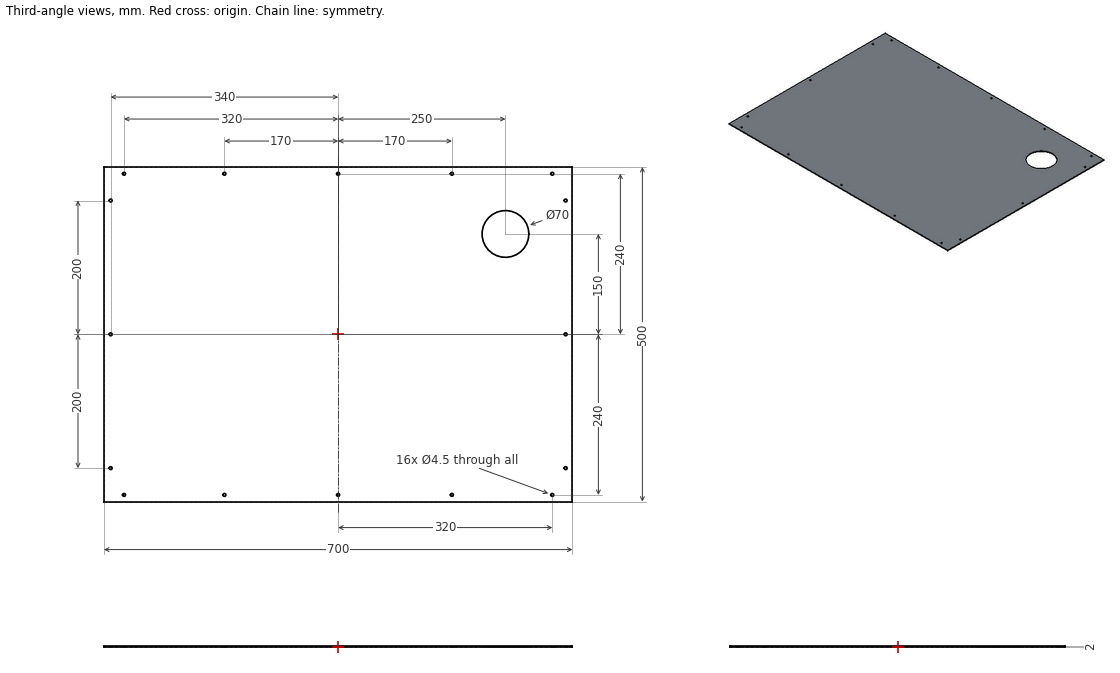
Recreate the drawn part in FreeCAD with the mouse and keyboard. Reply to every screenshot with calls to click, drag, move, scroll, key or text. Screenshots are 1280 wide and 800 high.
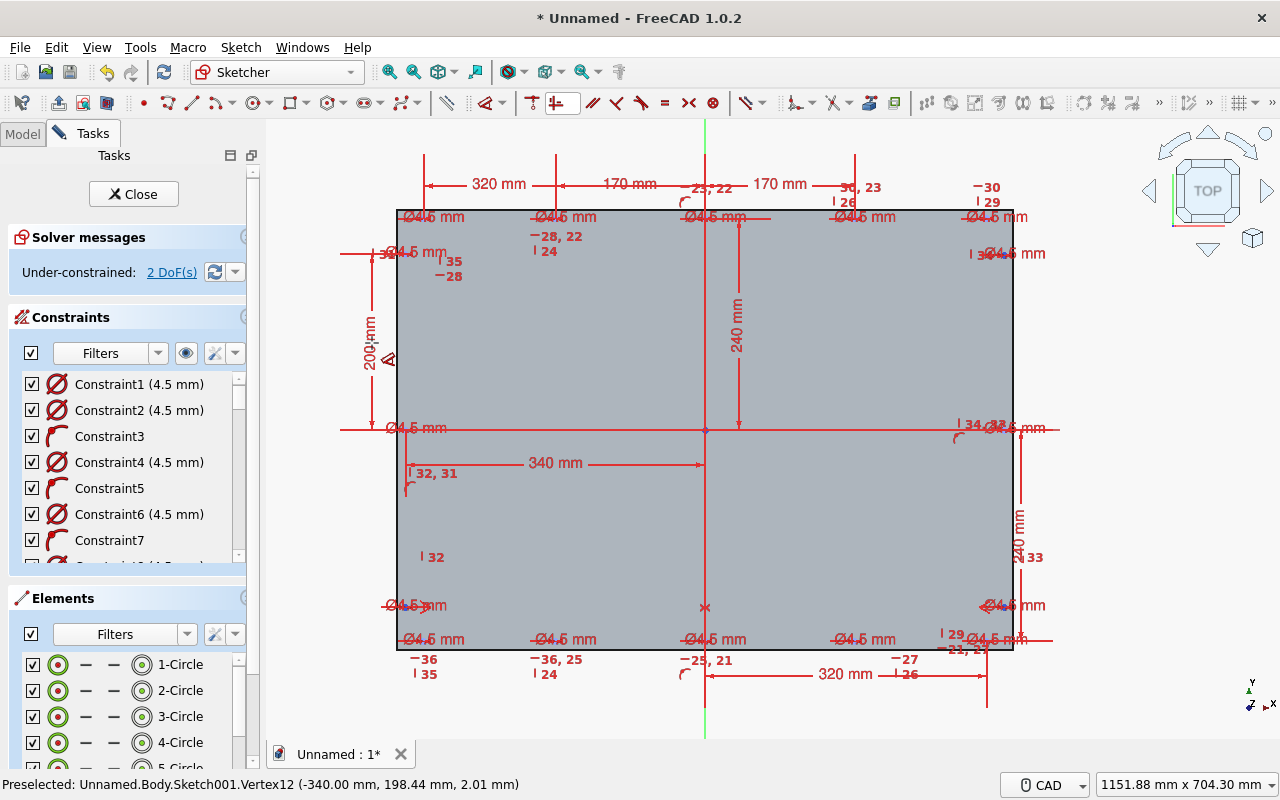
click(406, 607)
click(372, 519)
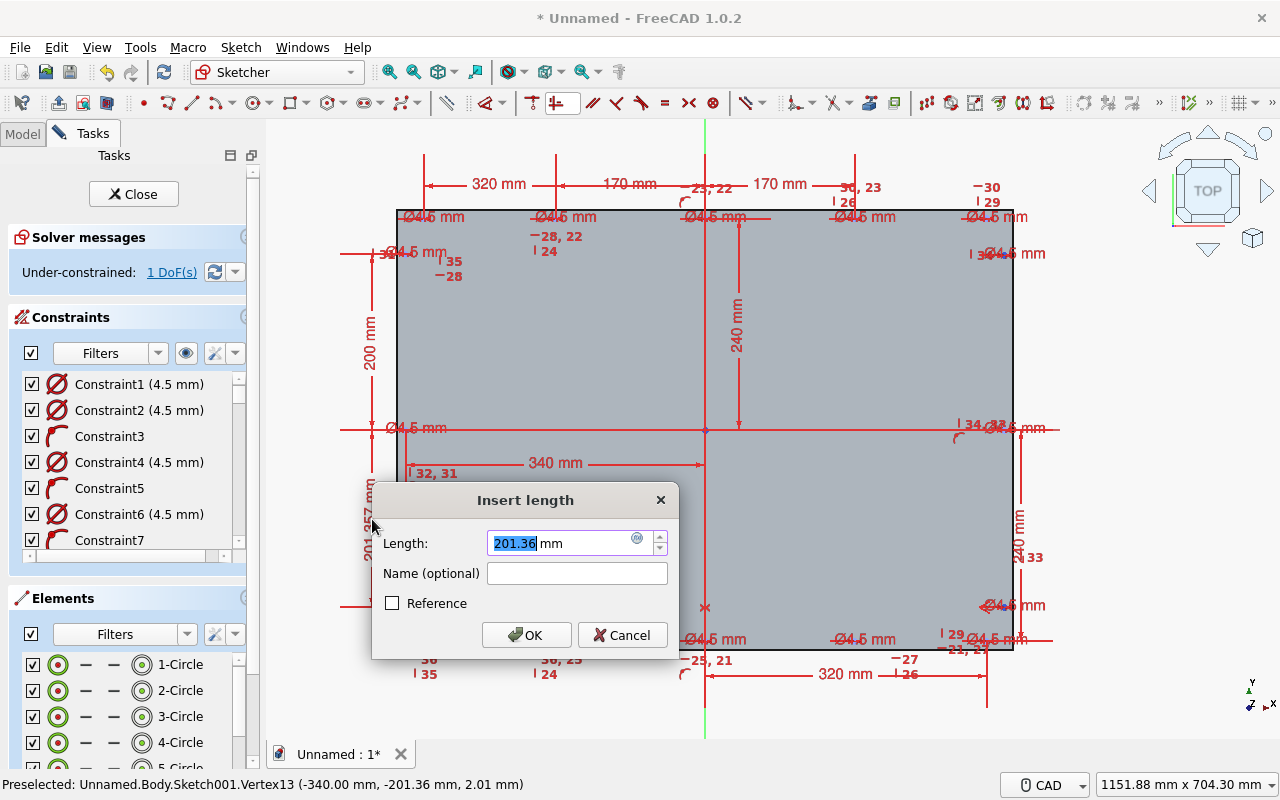
text(200)
key(Return)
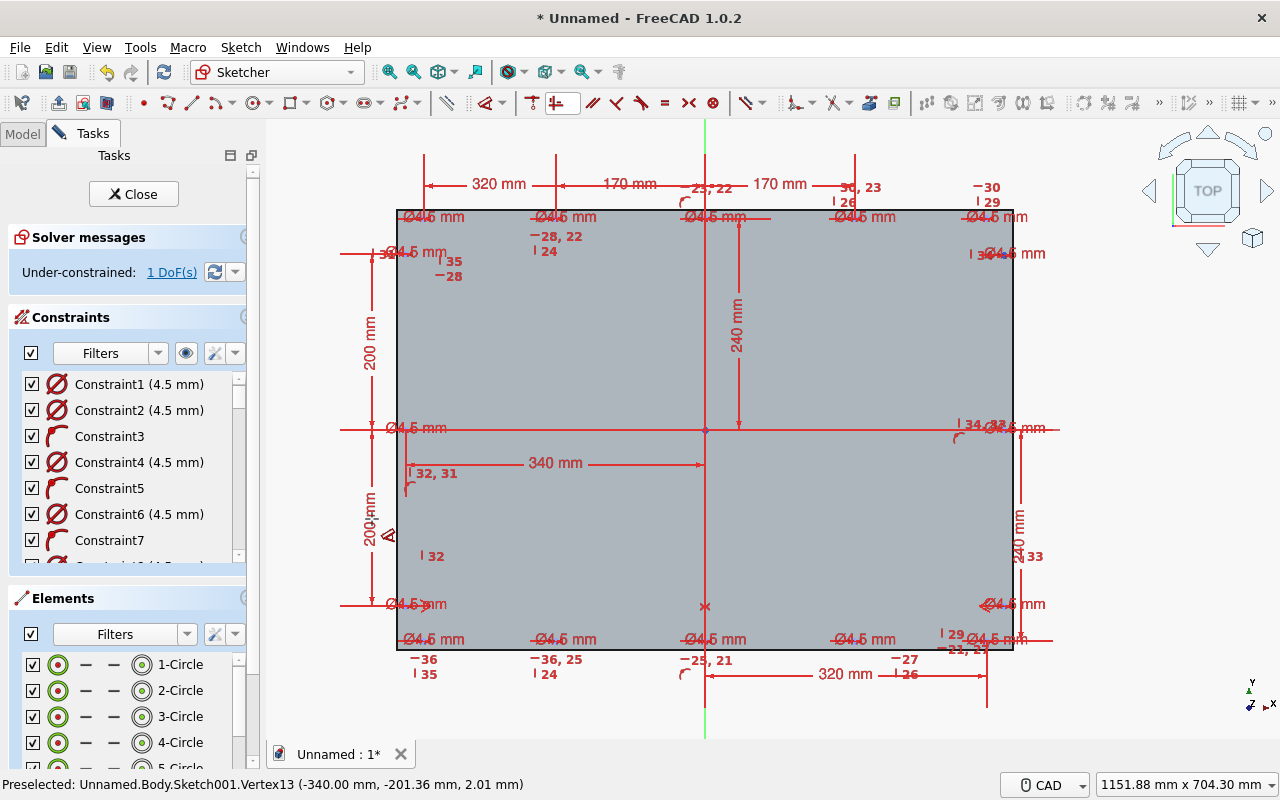
click(1005, 255)
click(1039, 343)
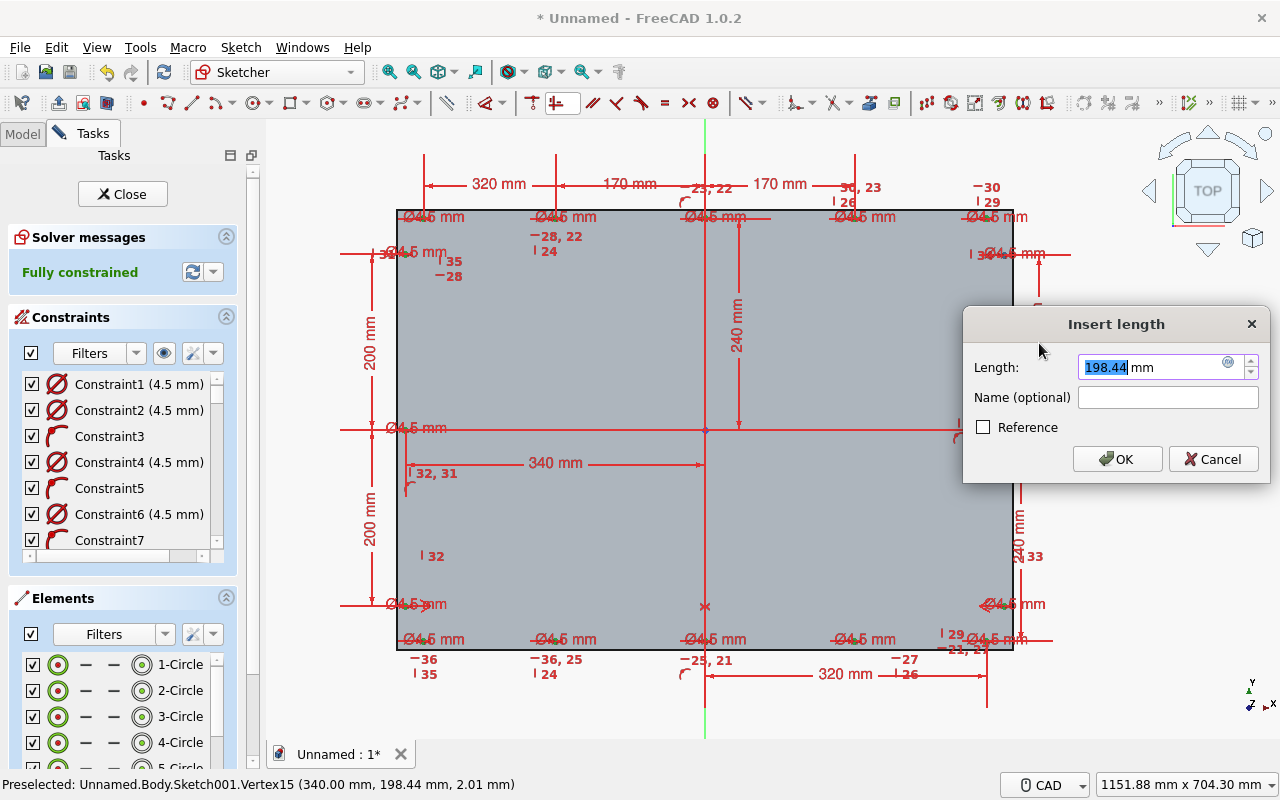
text(200)
key(Return)
key(Escape)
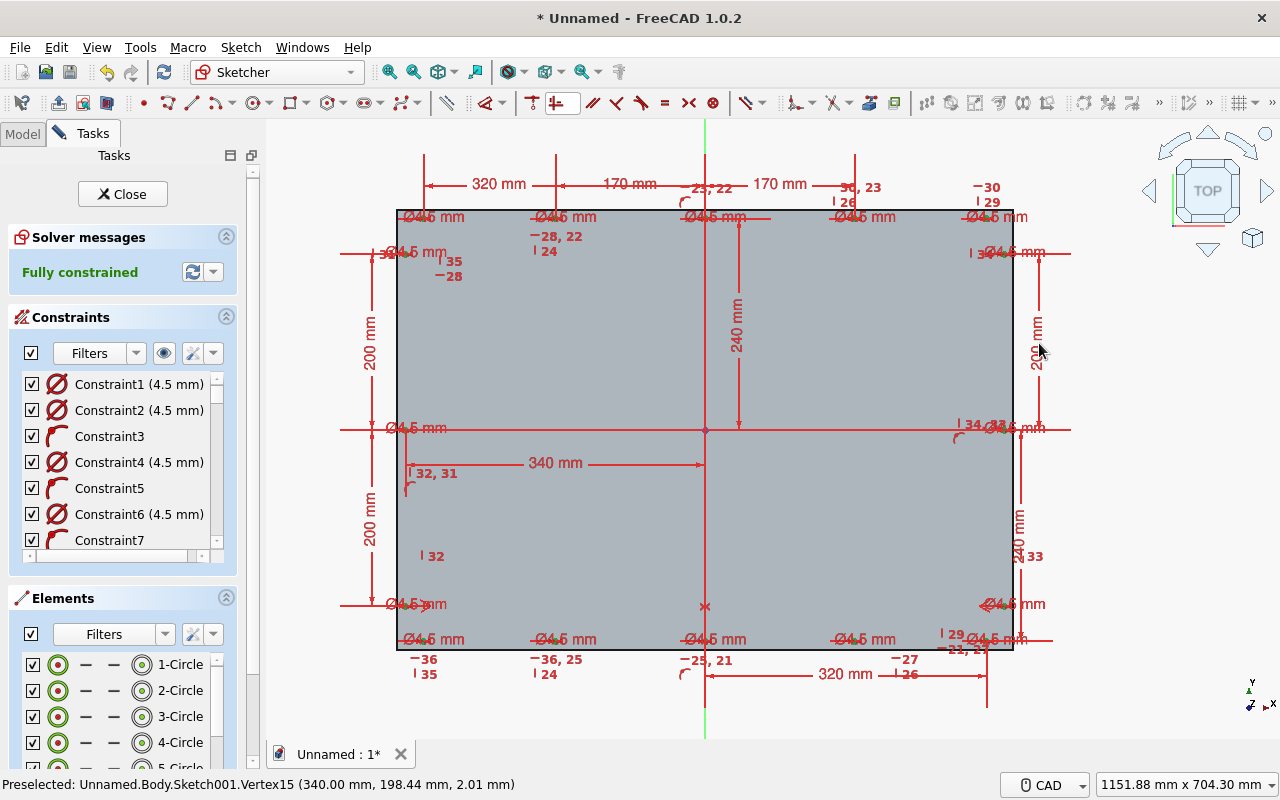
click(123, 194)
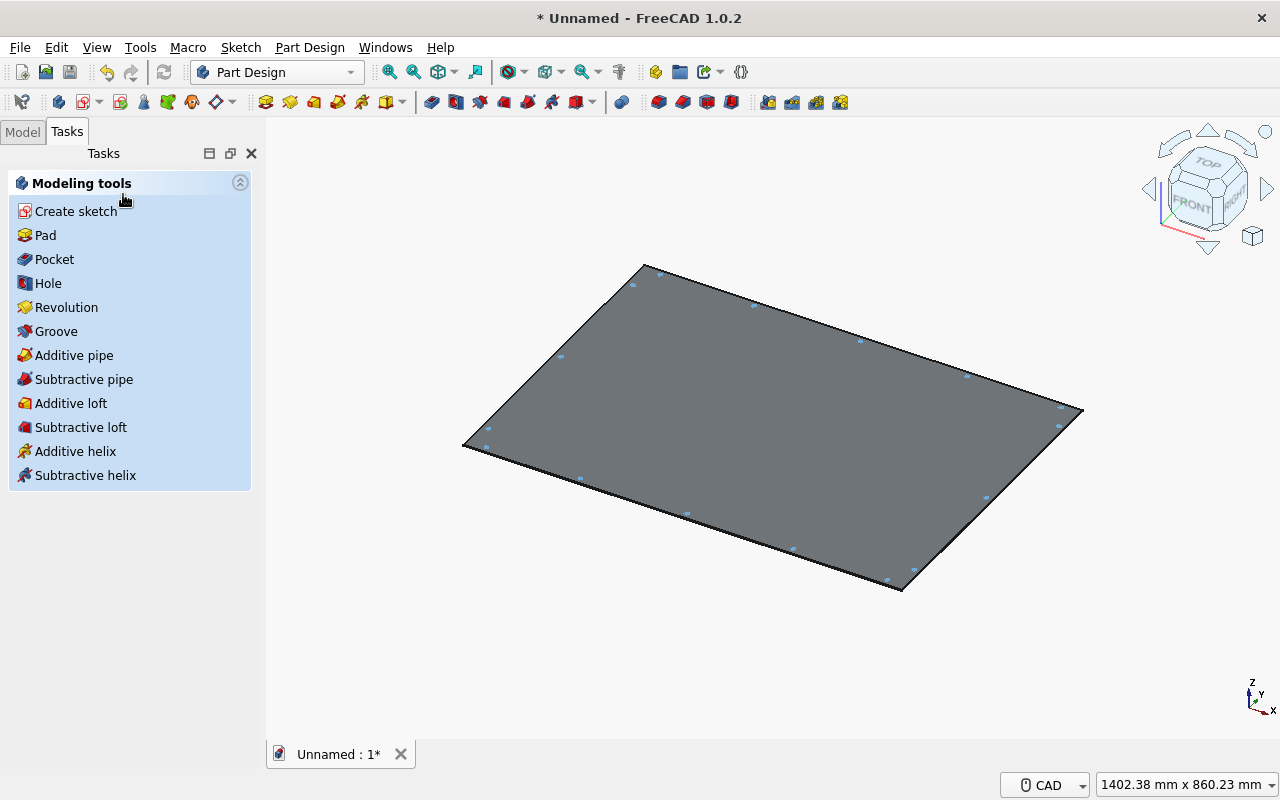
click(456, 102)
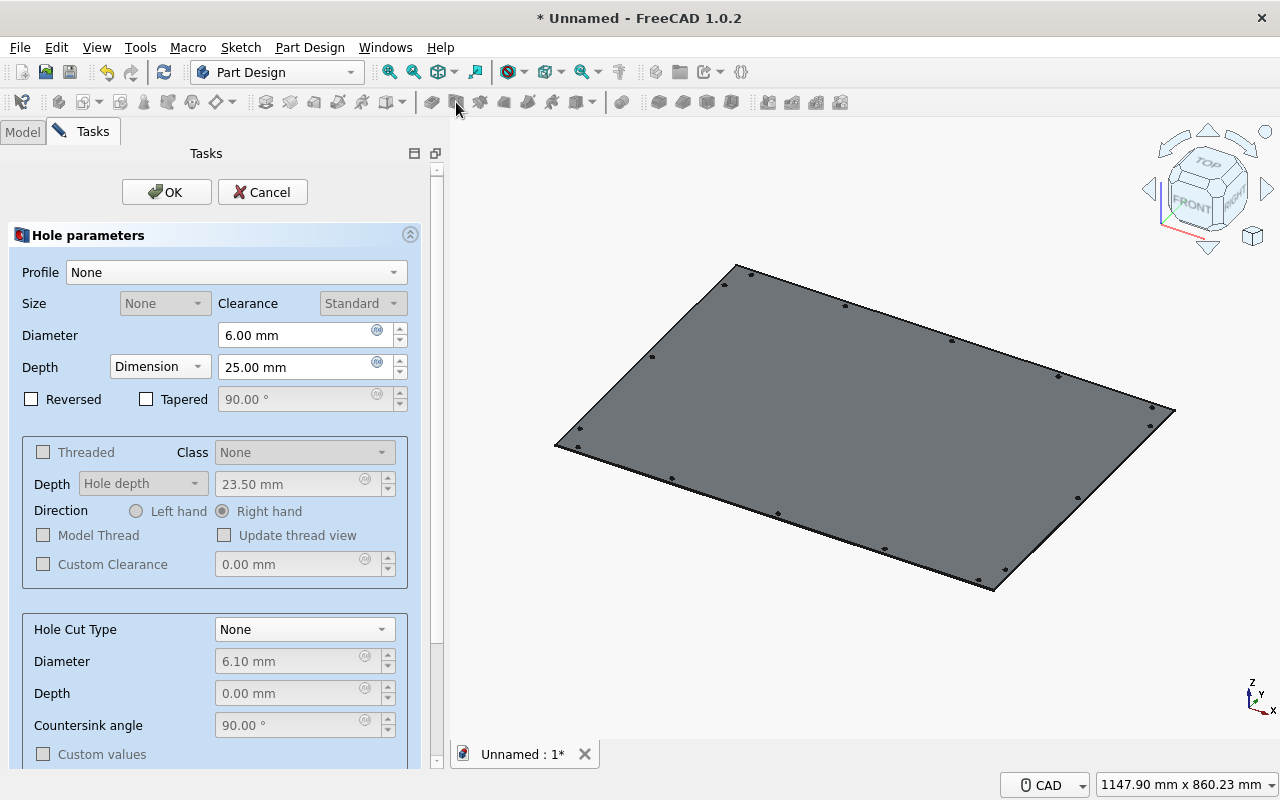
triple_click(305, 335)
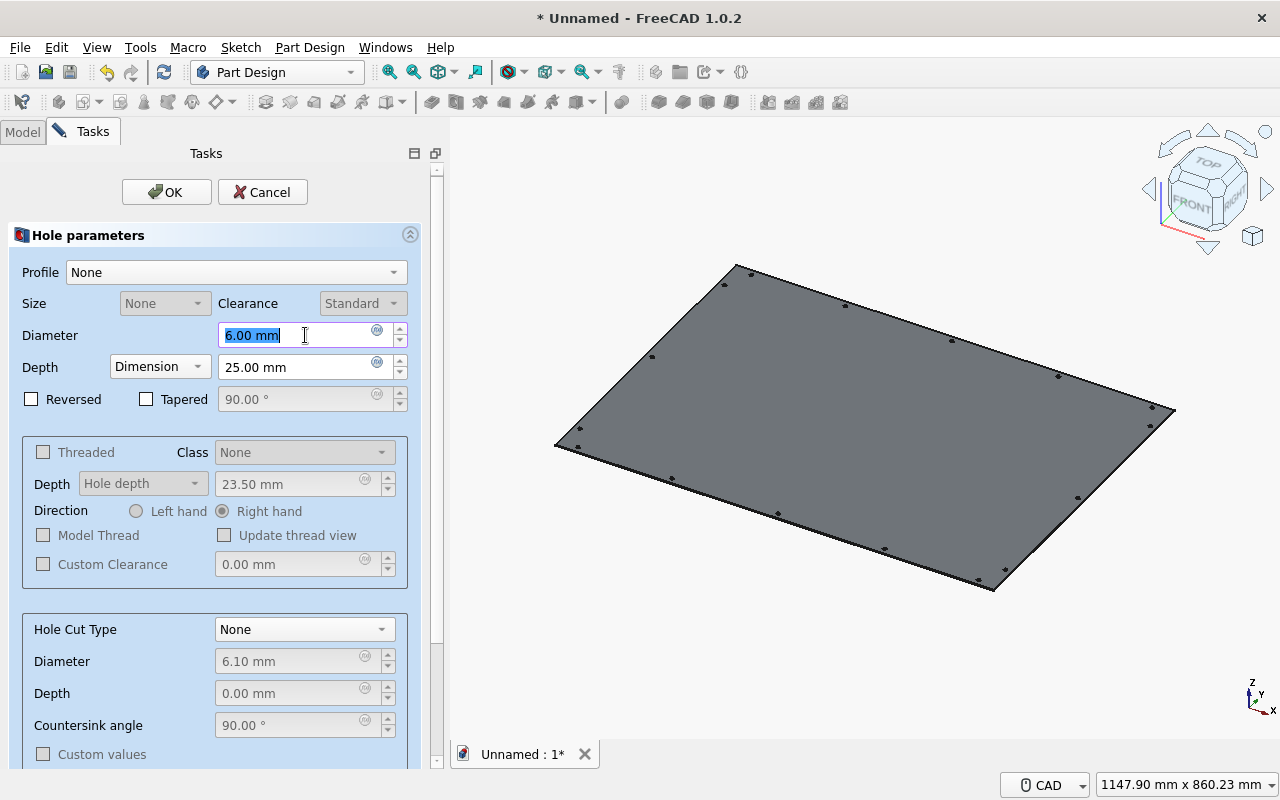
text(4.5)
key(Tab)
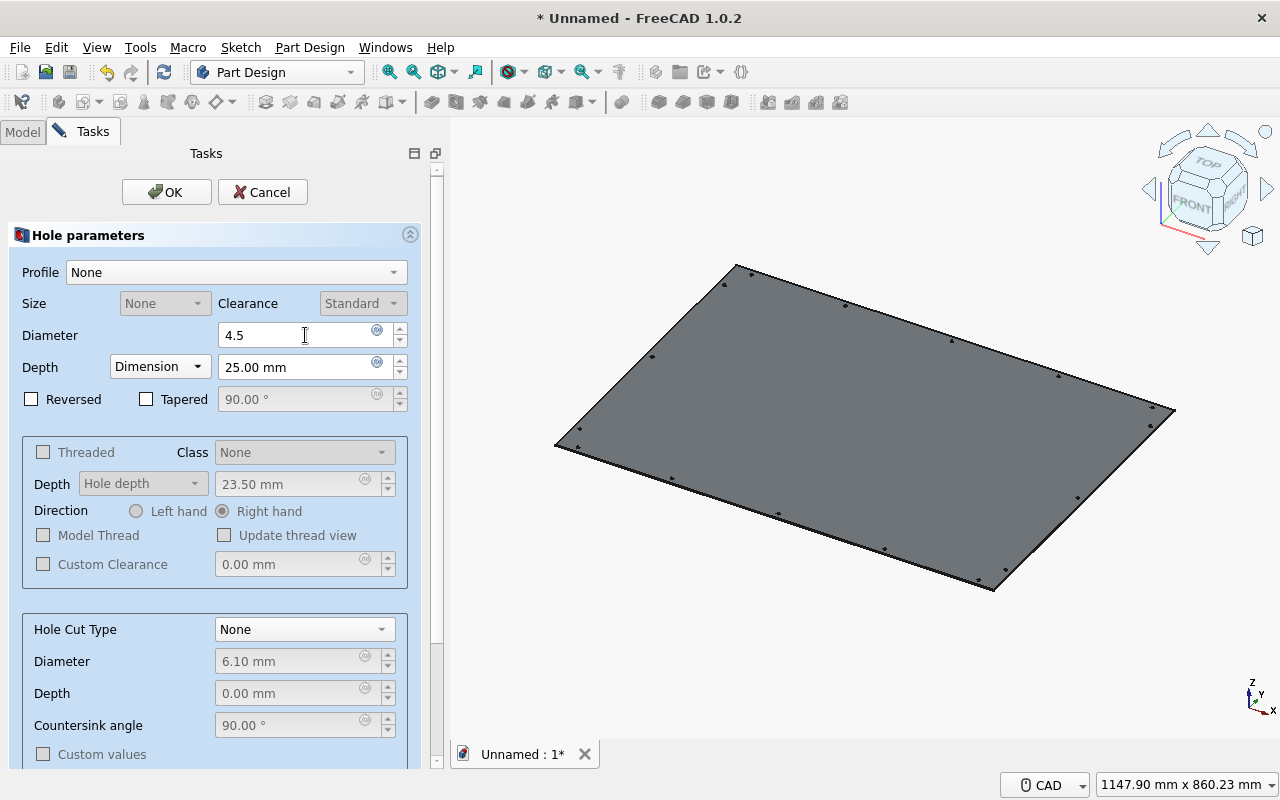
click(161, 366)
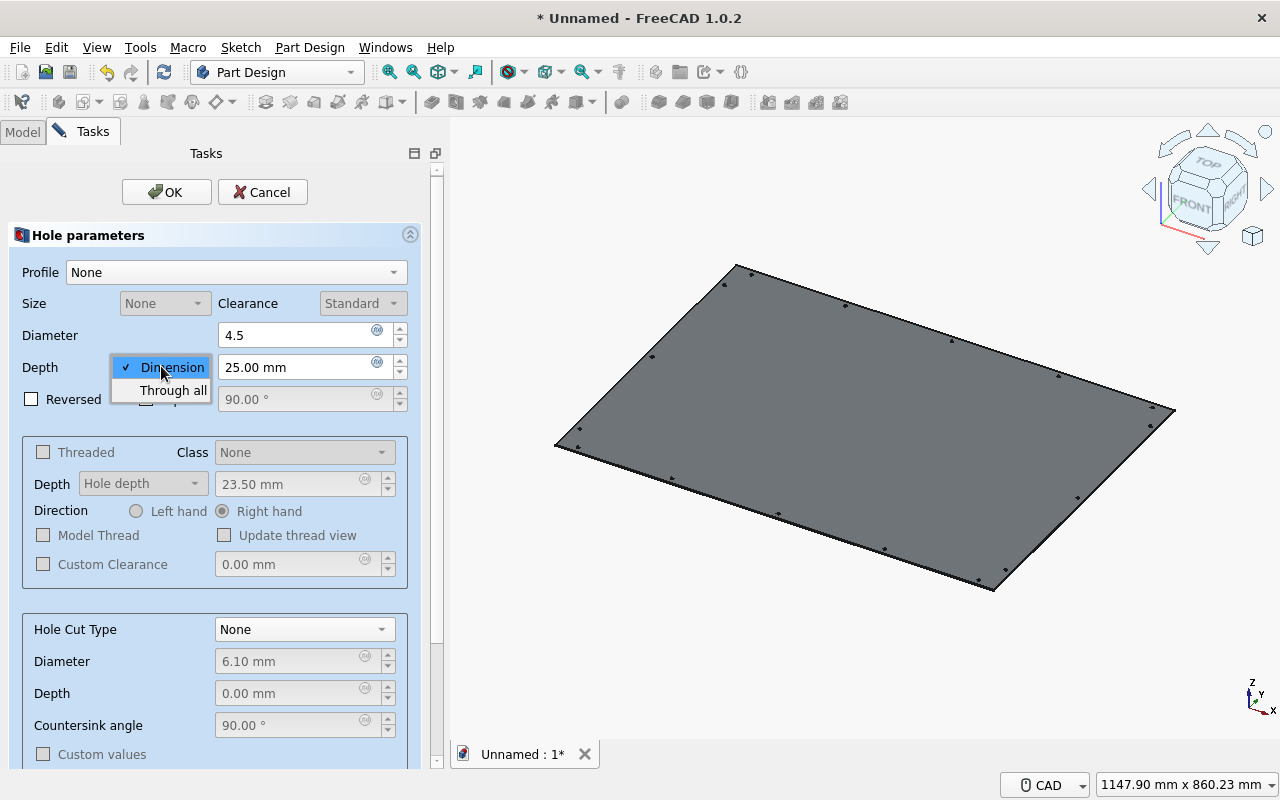
click(160, 390)